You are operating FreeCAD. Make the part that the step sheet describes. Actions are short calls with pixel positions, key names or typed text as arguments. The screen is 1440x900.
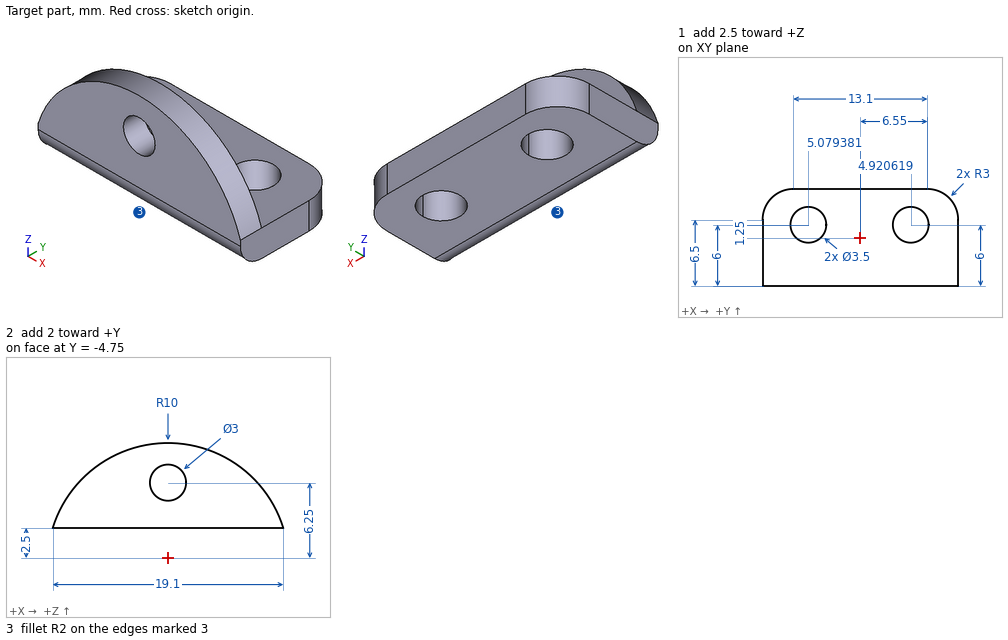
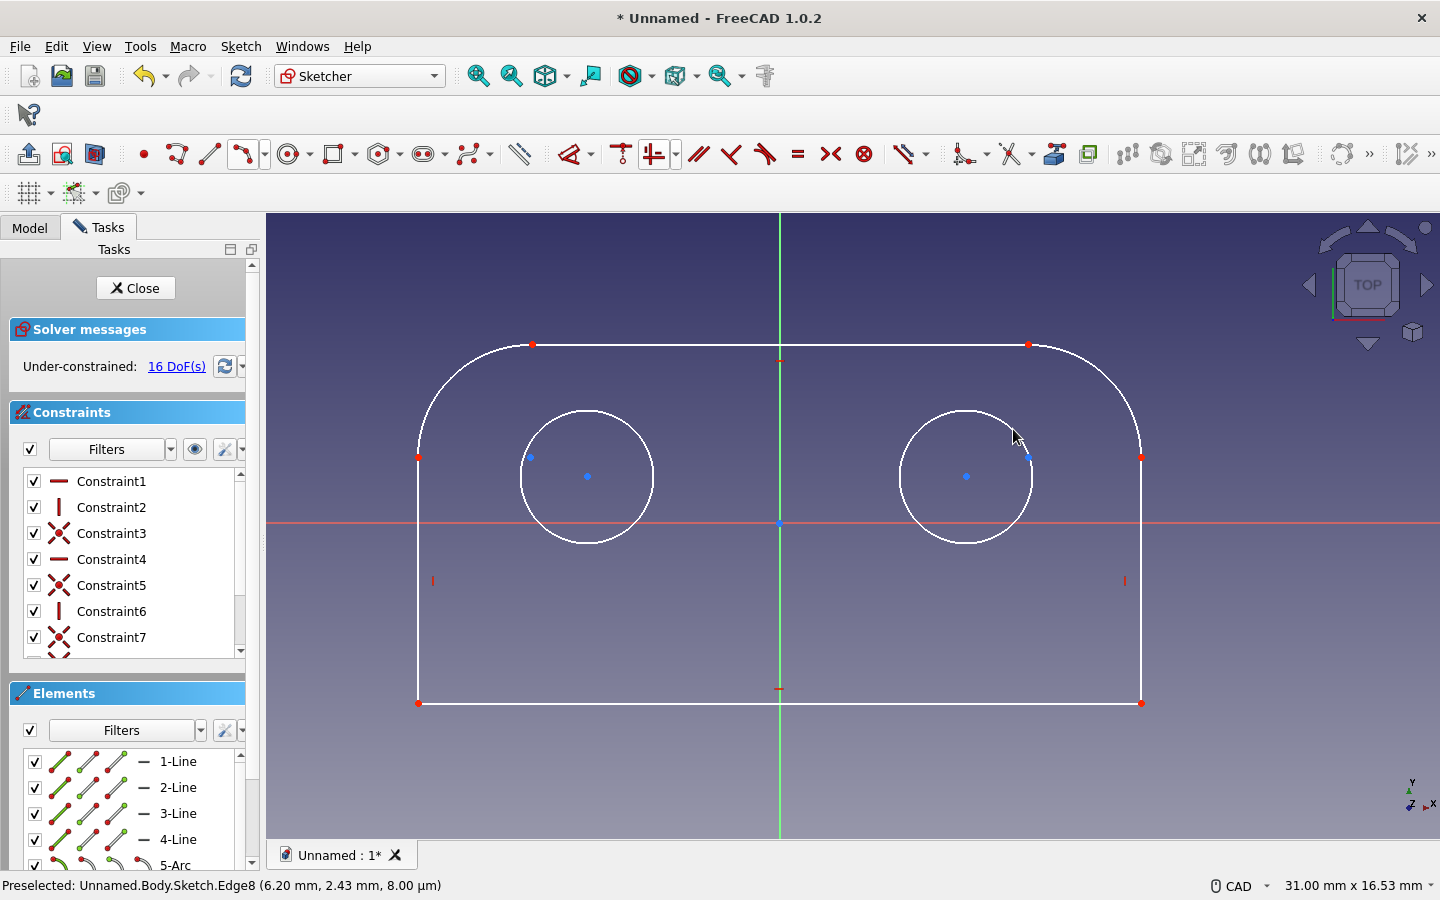
click(879, 345)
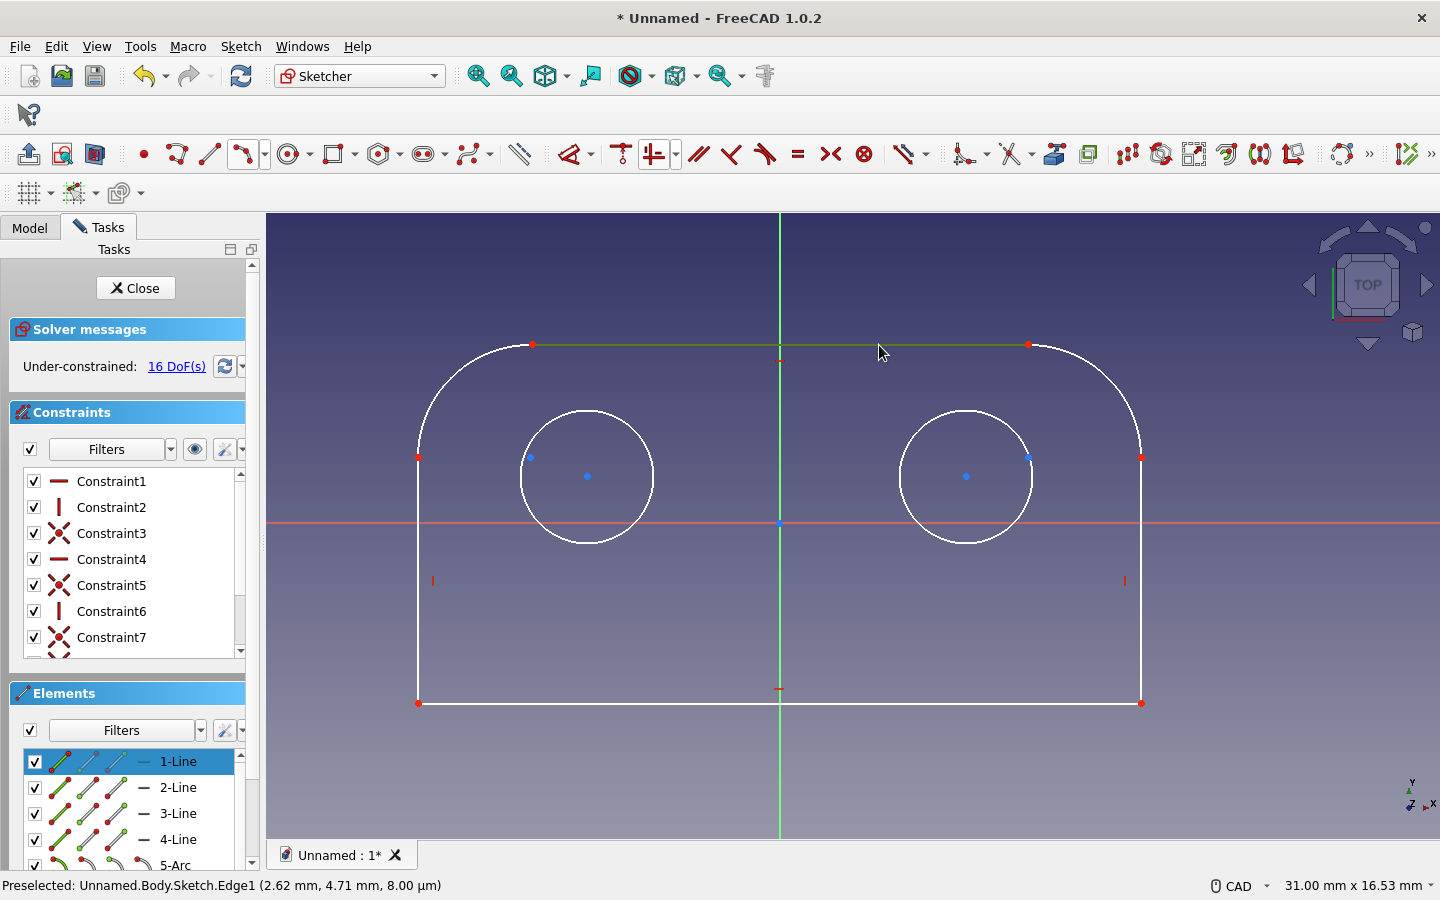
click(480, 357)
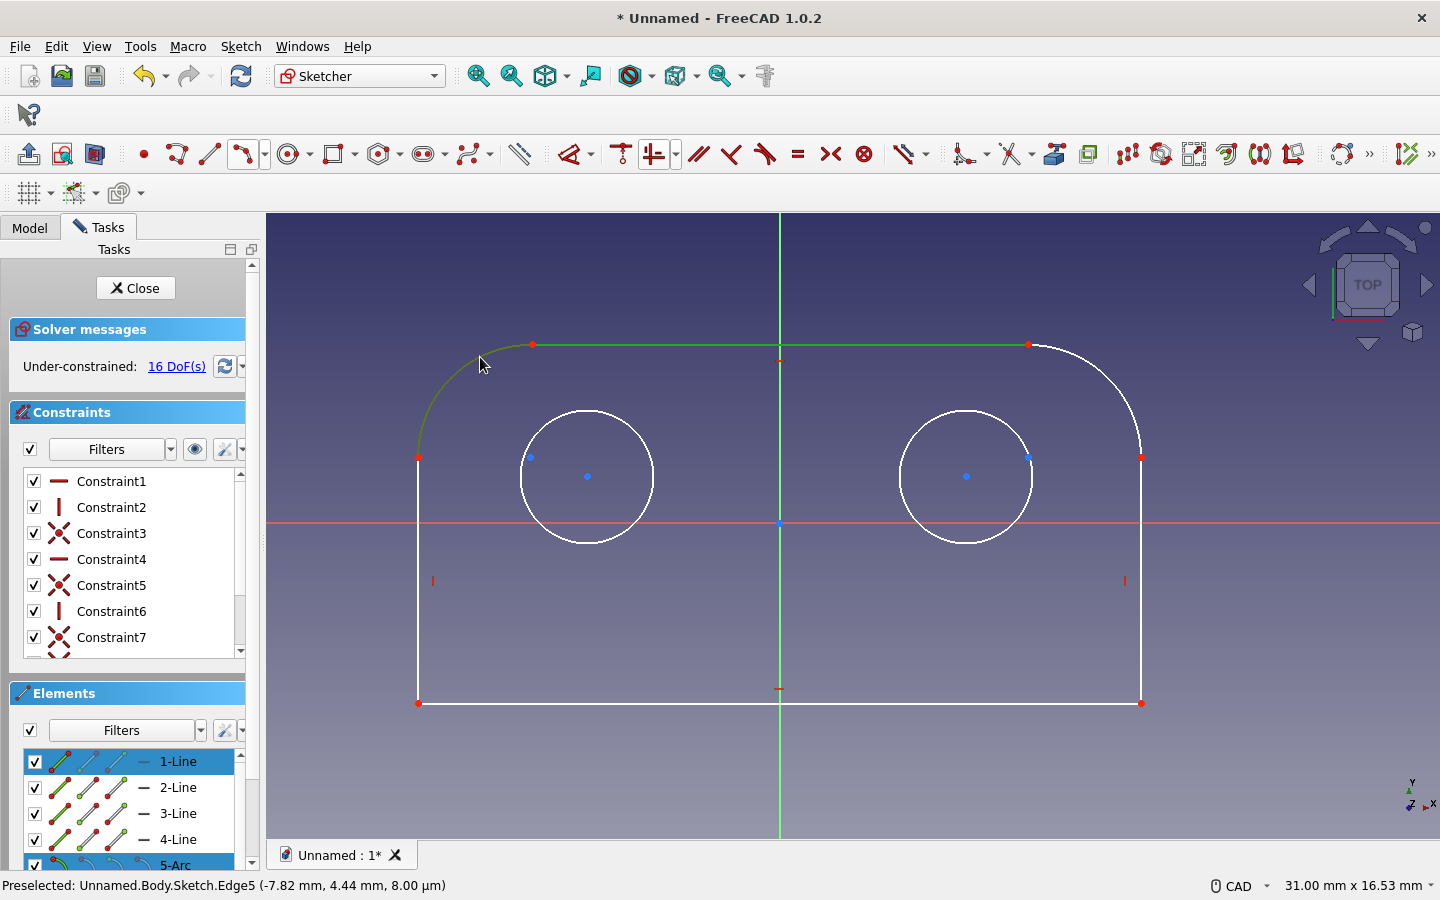
click(765, 154)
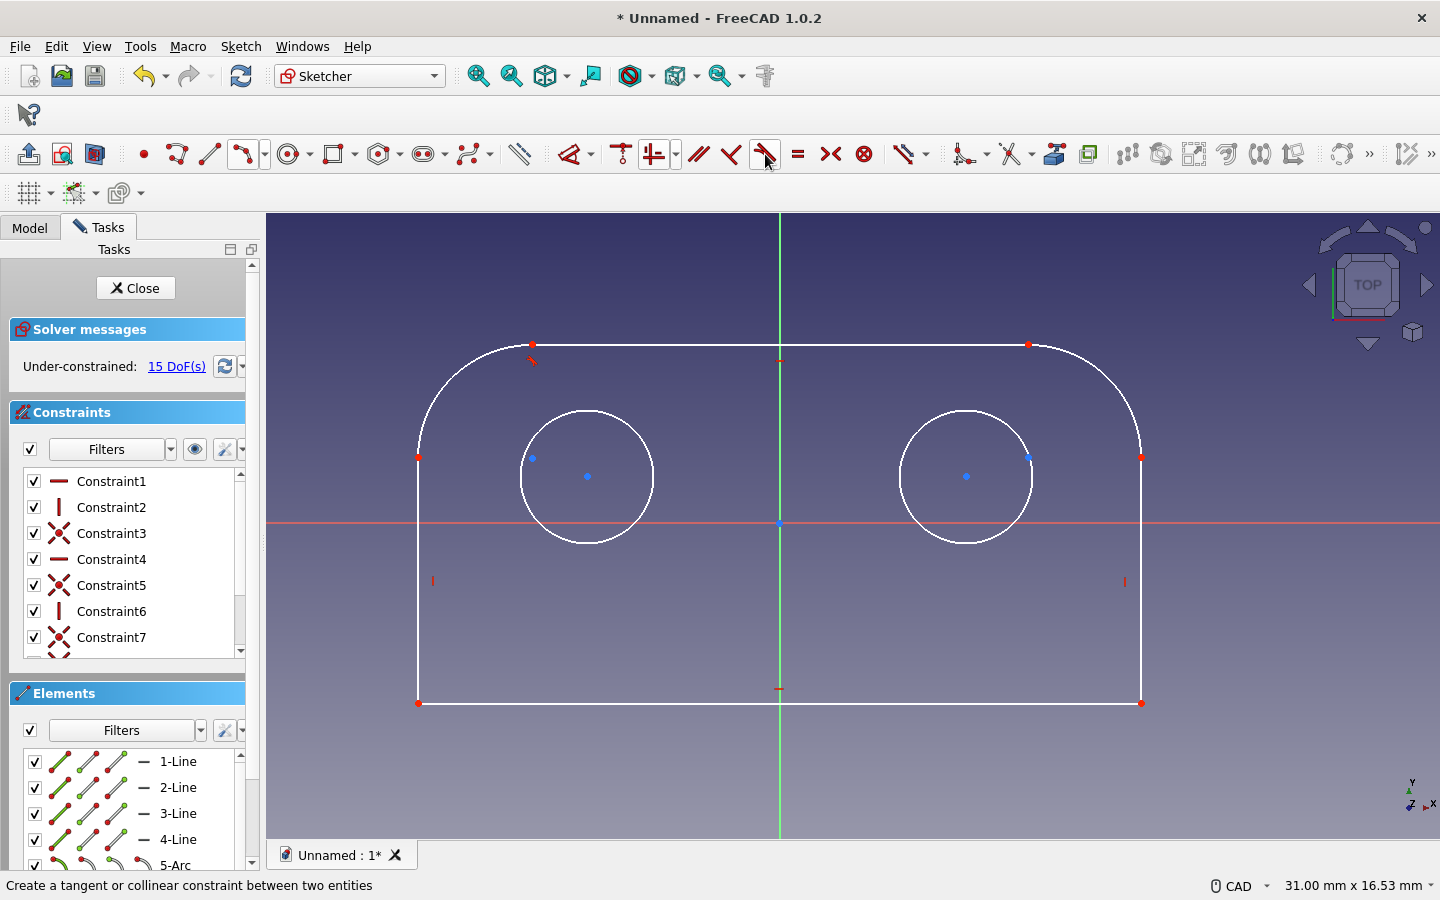
click(879, 345)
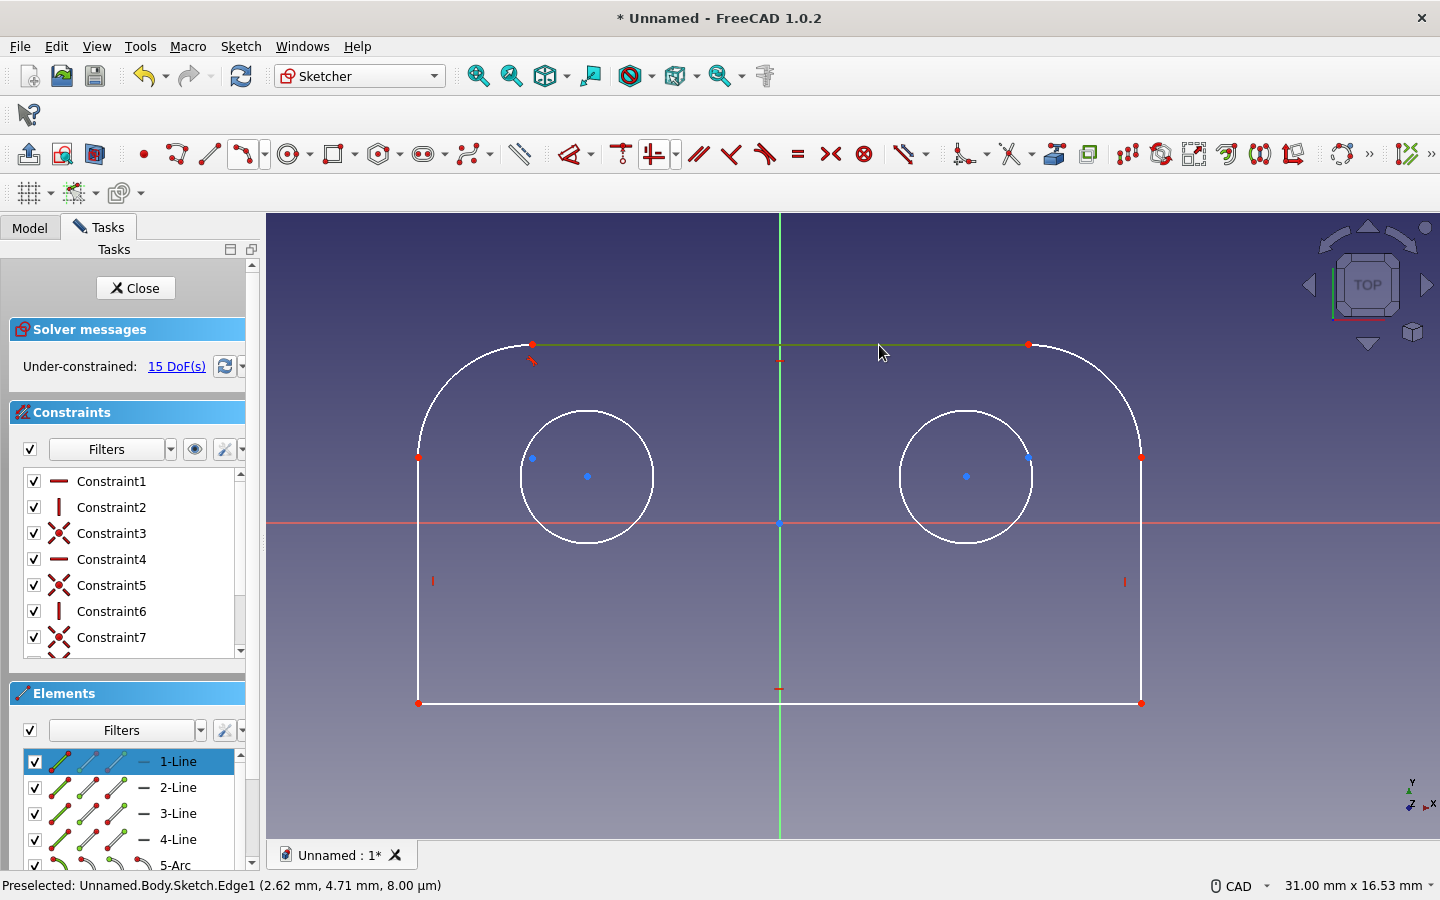
click(1129, 407)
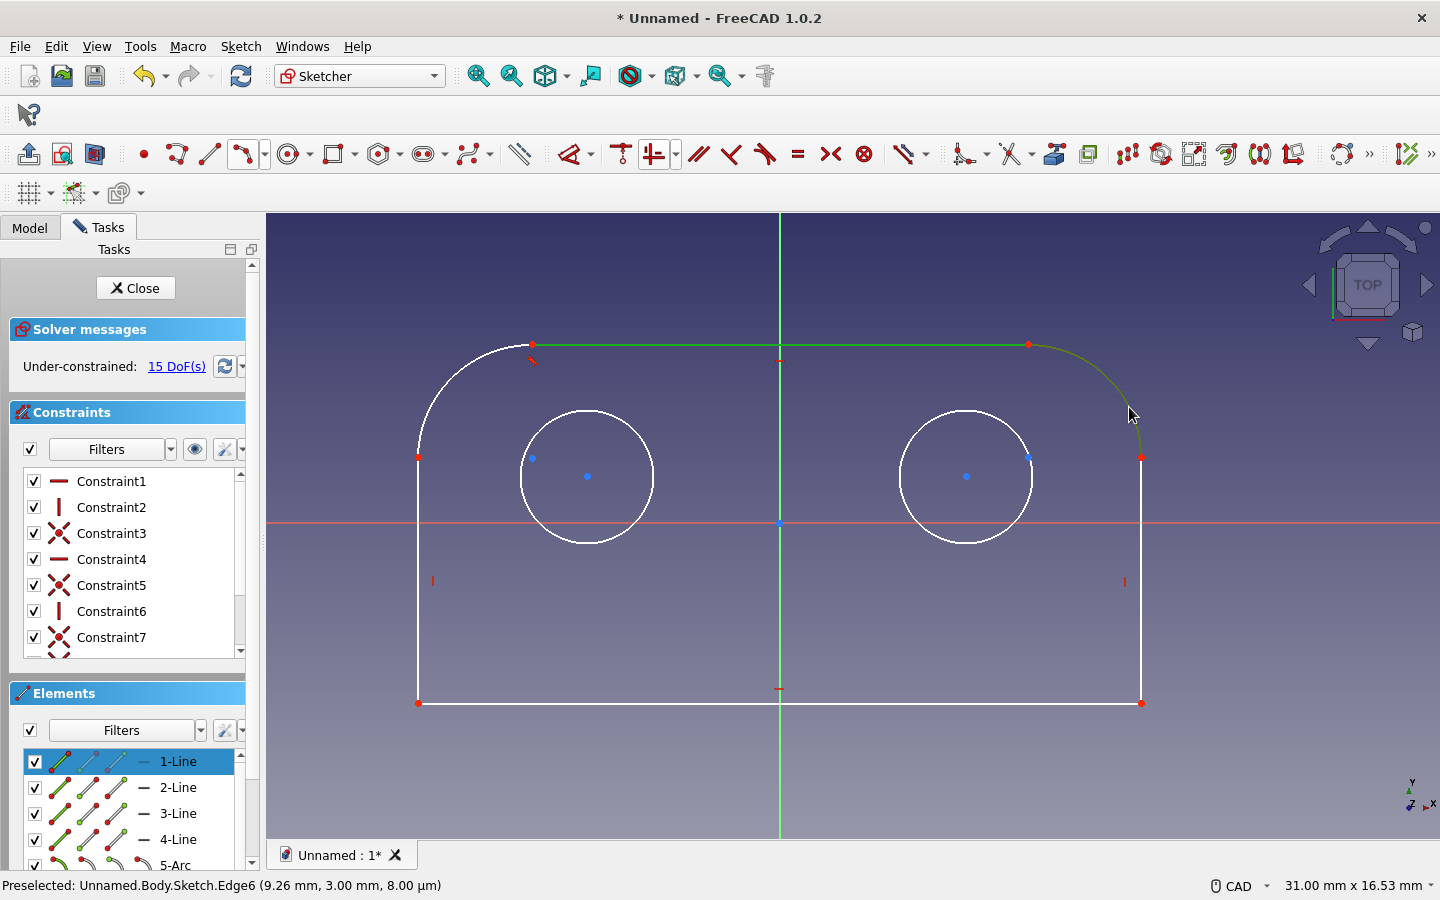
click(765, 154)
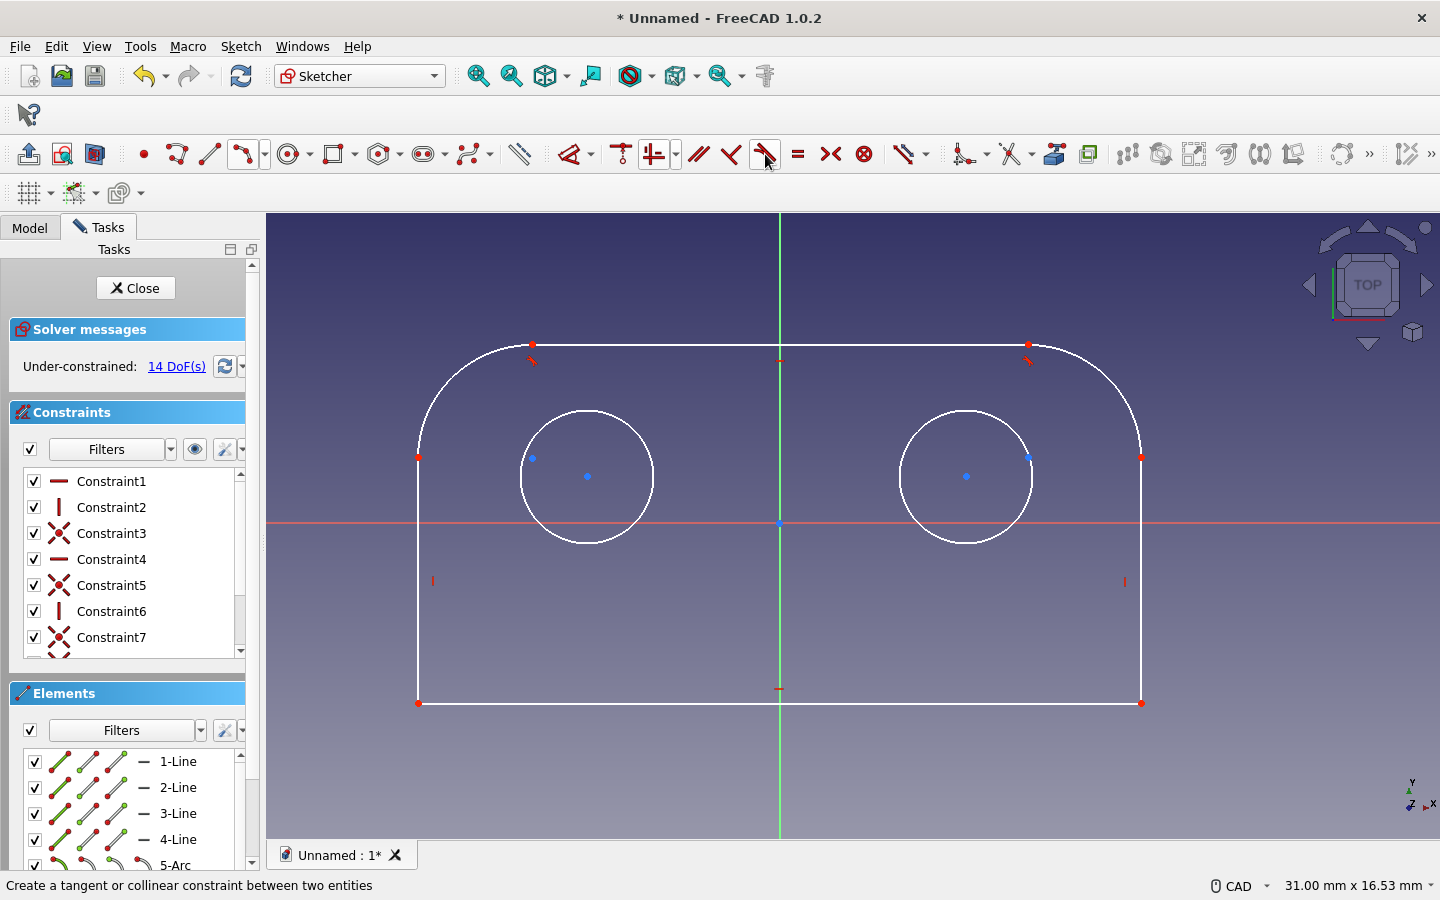
click(418, 630)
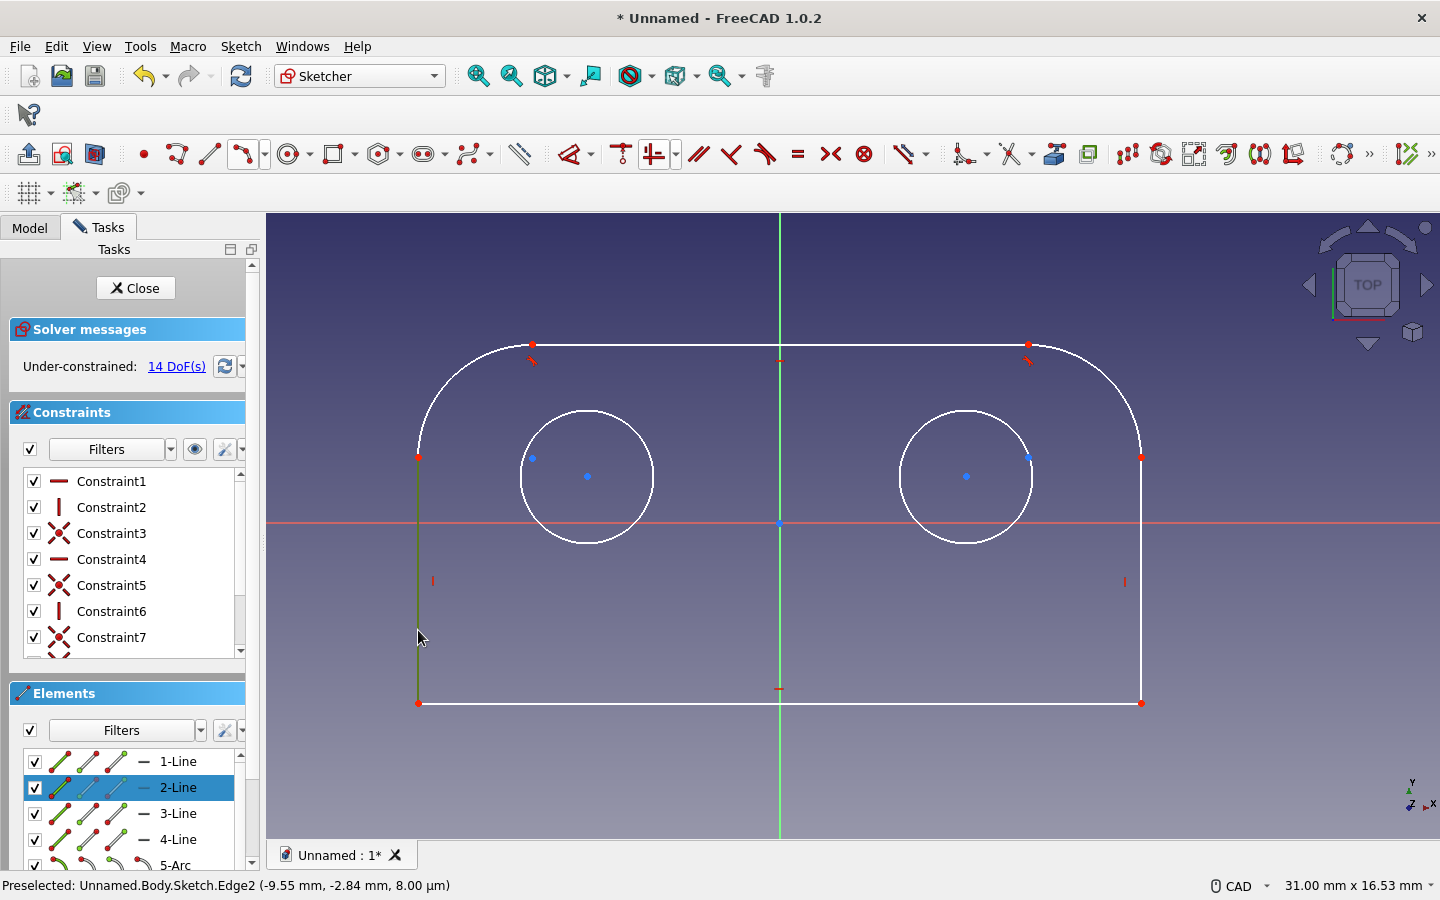
click(481, 357)